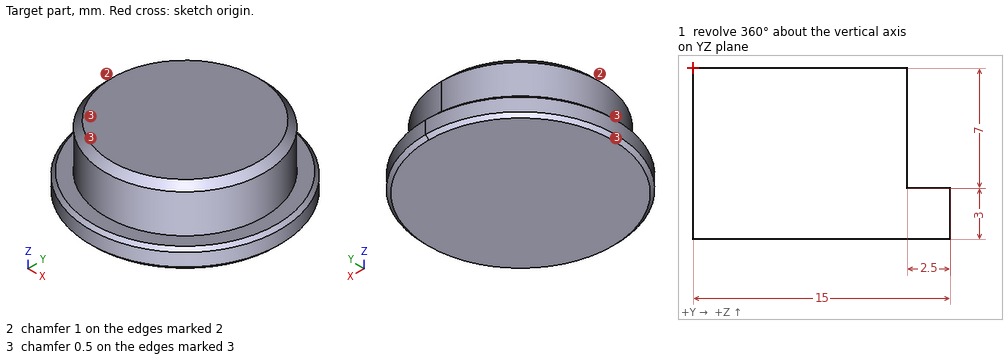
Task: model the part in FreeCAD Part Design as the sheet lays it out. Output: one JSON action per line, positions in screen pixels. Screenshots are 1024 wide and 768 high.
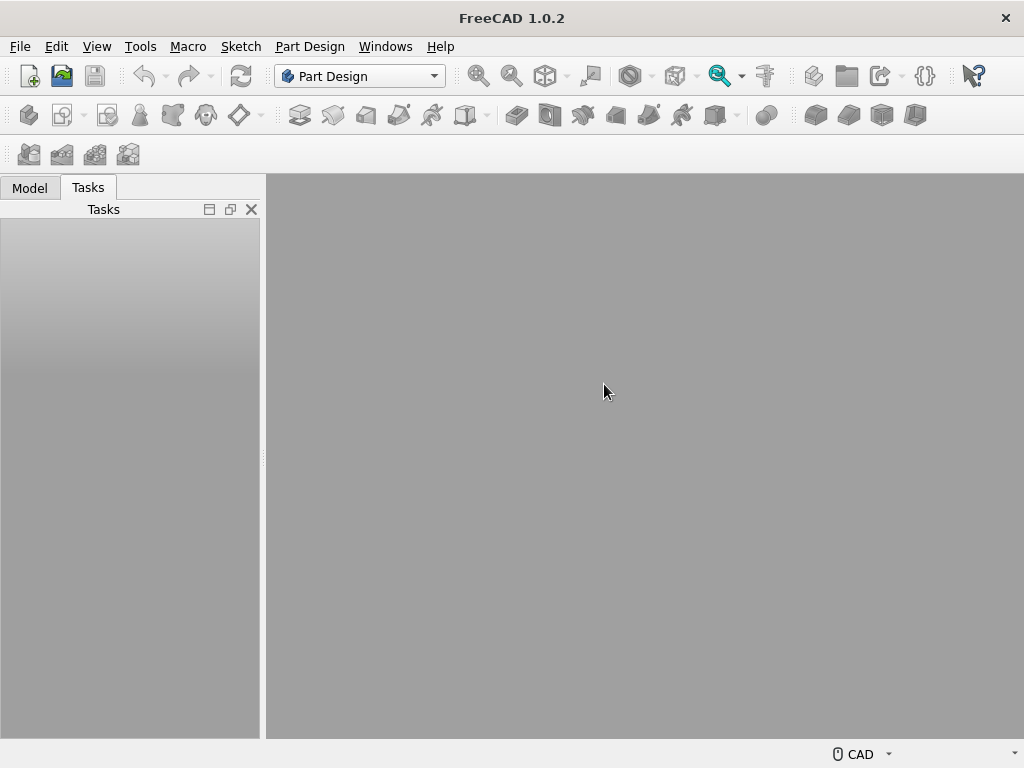
{"action": "left_click", "coordinate": [29, 76]}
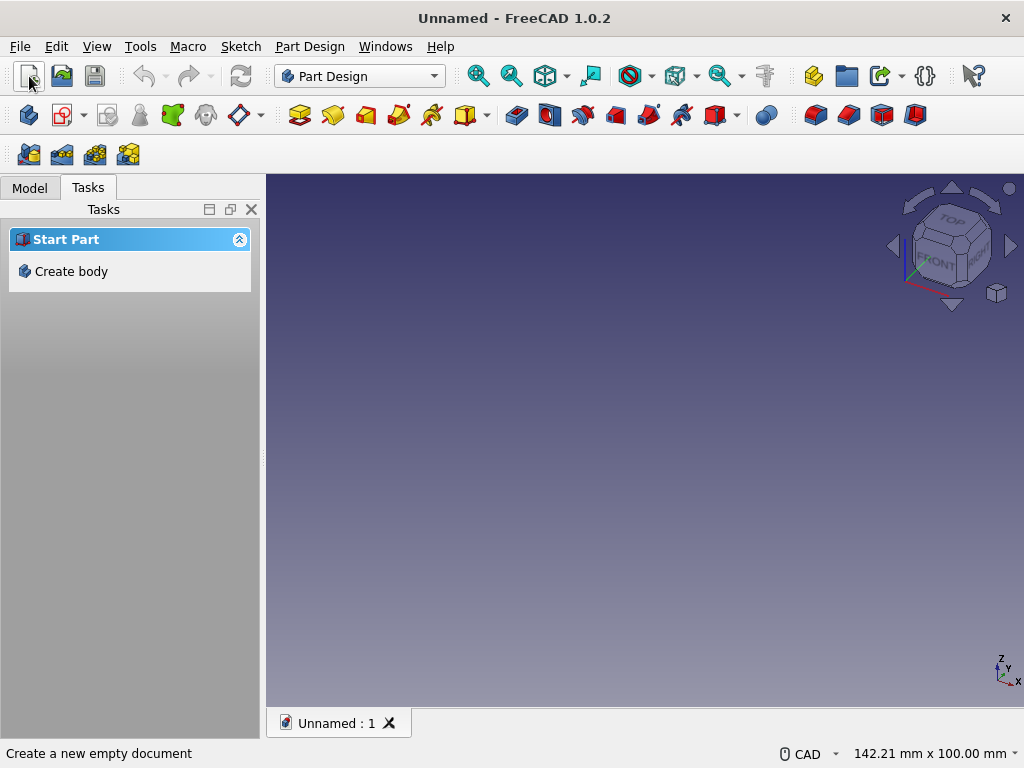
{"action": "left_click", "coordinate": [62, 116]}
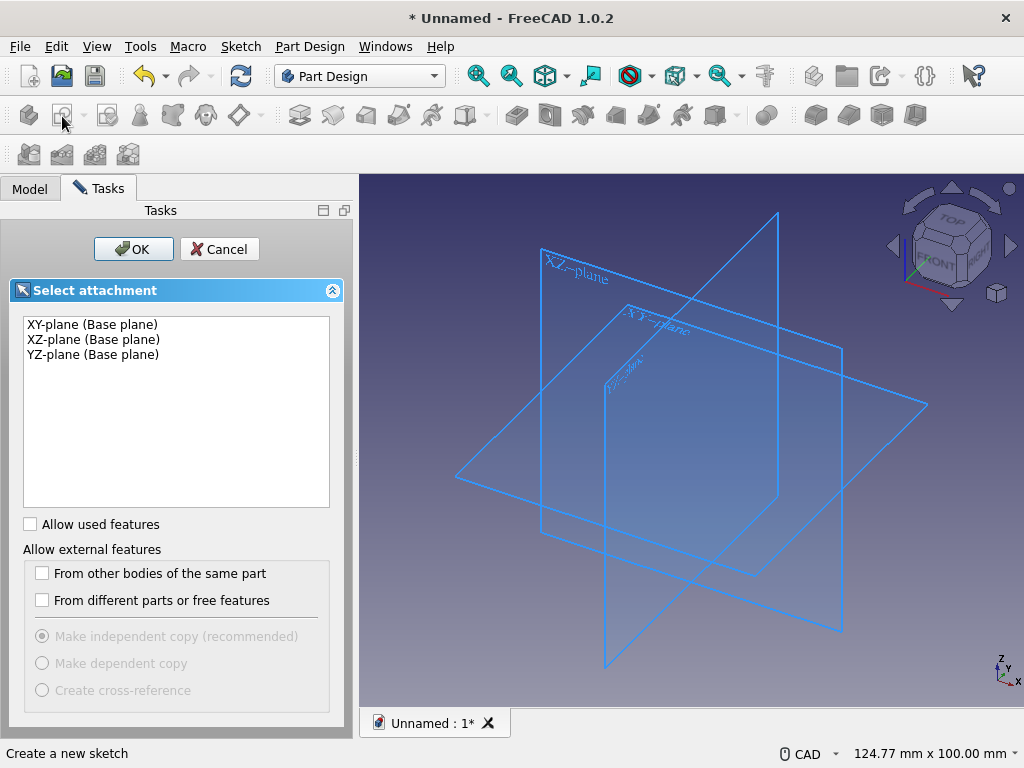
{"action": "left_click", "coordinate": [84, 354]}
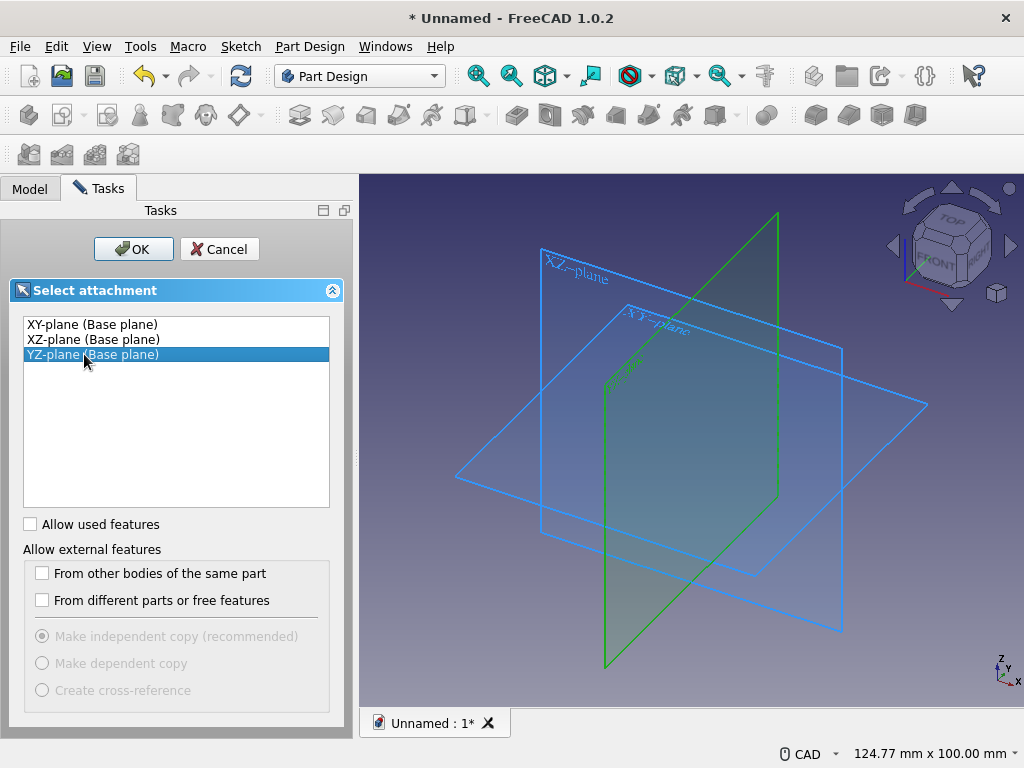
{"action": "left_click", "coordinate": [134, 249]}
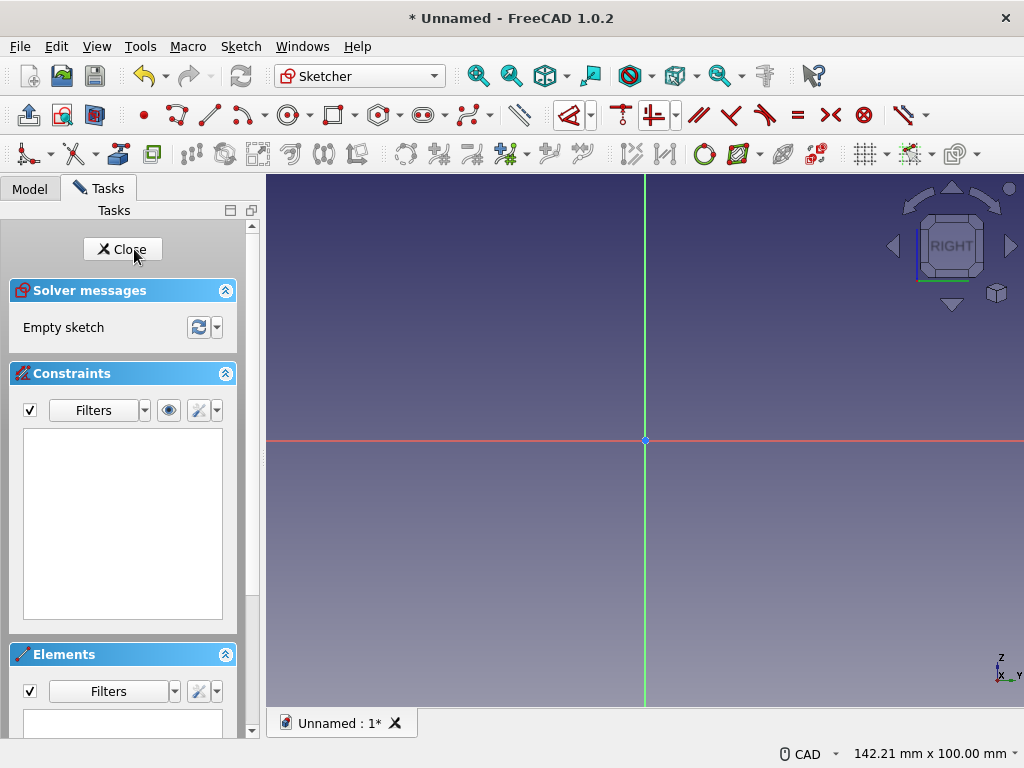
{"action": "scroll", "coordinate": [712, 474], "scroll_direction": "up", "scroll_amount": 8}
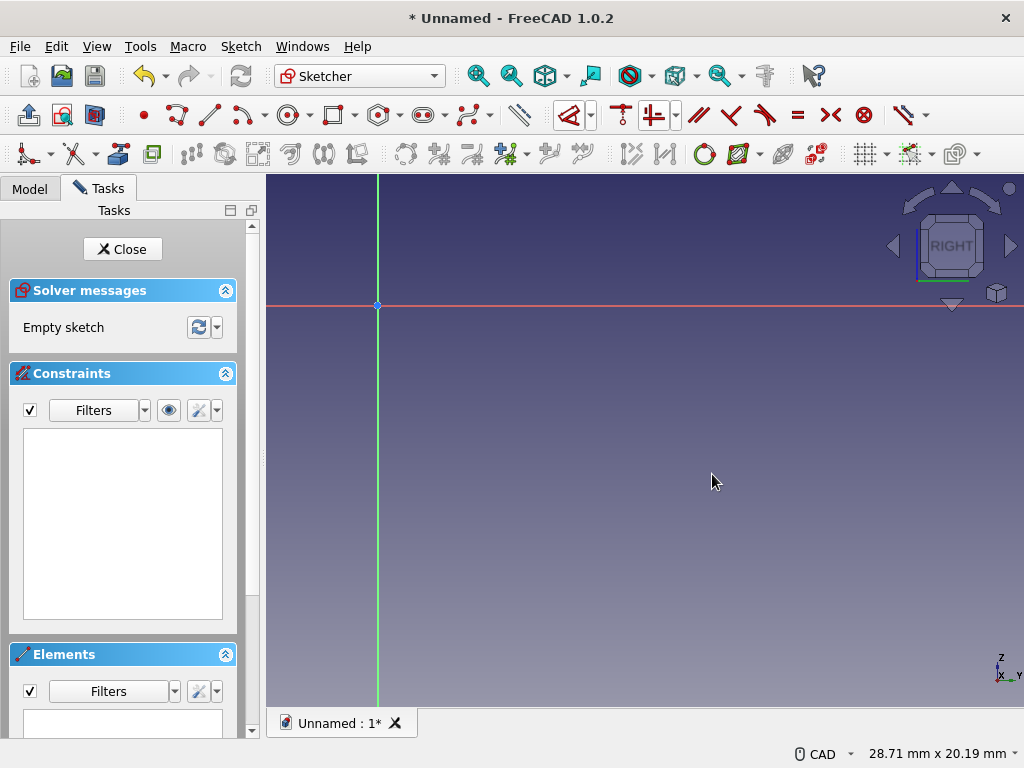
{"action": "left_click", "coordinate": [177, 116]}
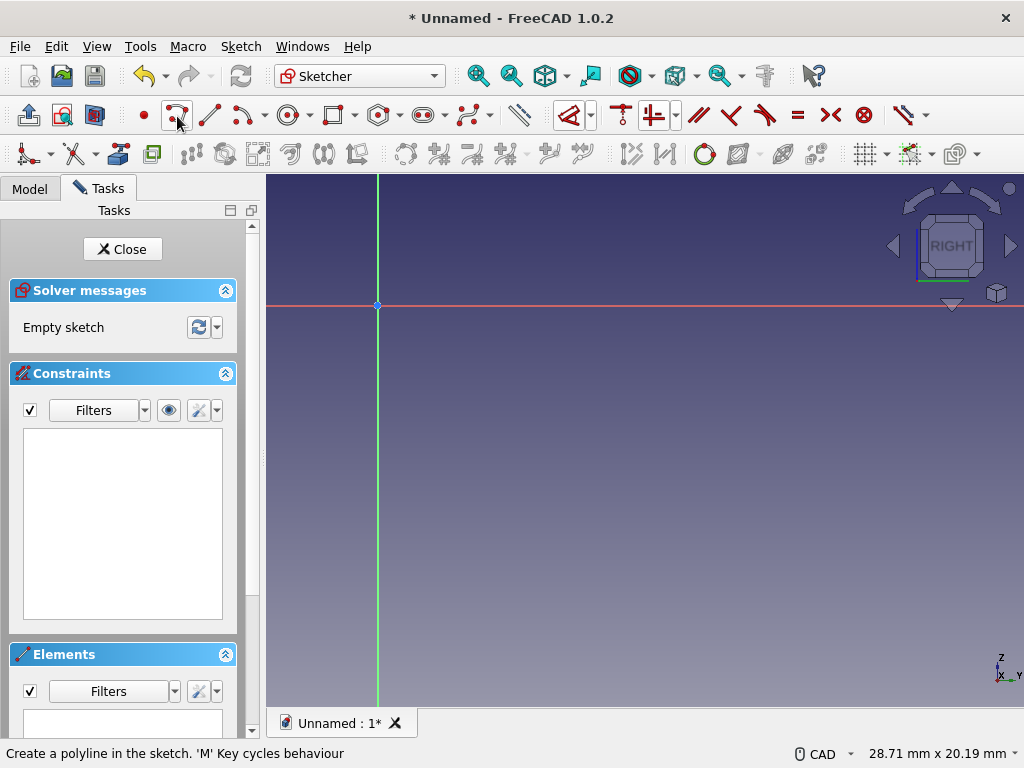
{"action": "left_click", "coordinate": [378, 306]}
{"action": "left_click", "coordinate": [387, 570]}
{"action": "left_click", "coordinate": [774, 570]}
{"action": "left_click", "coordinate": [774, 491]}
{"action": "left_click", "coordinate": [708, 491]}
{"action": "left_click", "coordinate": [708, 315]}
{"action": "left_click", "coordinate": [378, 306]}
{"action": "key", "text": "Escape"}
{"action": "key", "text": "Escape"}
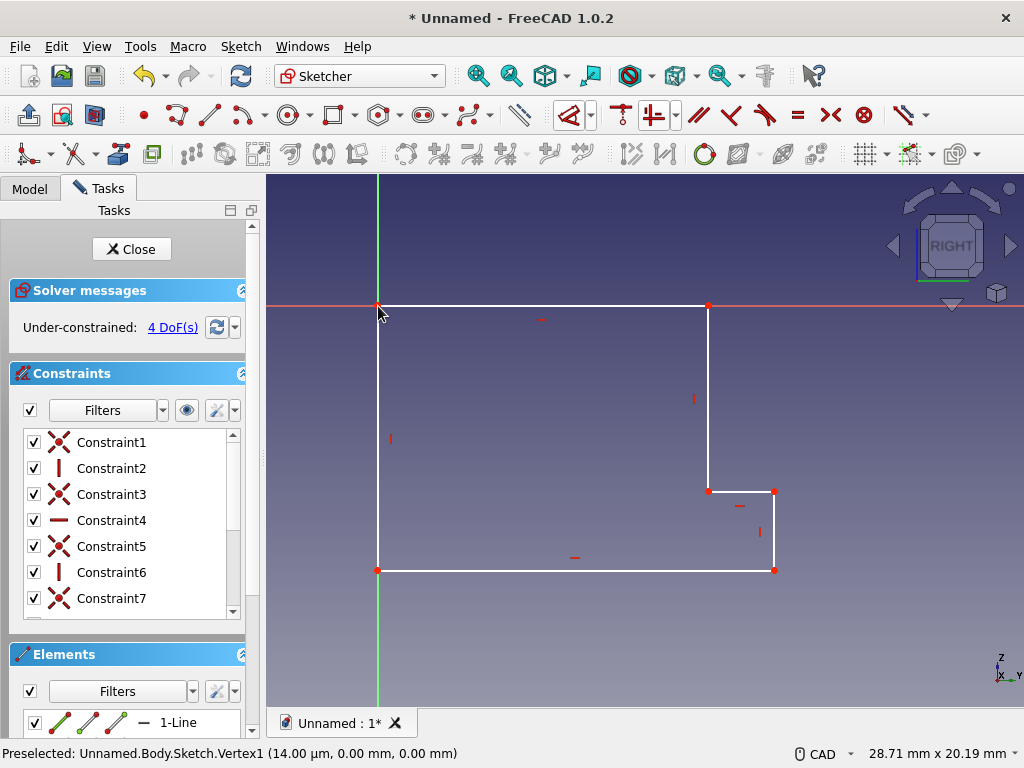
{"action": "left_click", "coordinate": [568, 116]}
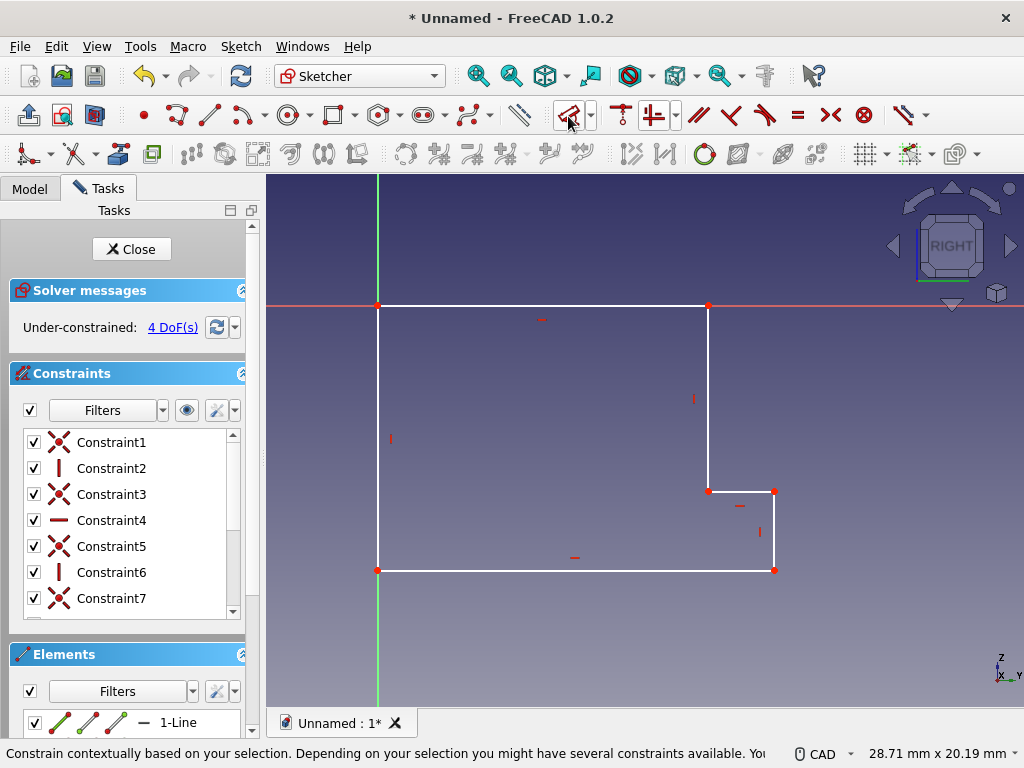
{"action": "left_click", "coordinate": [774, 547]}
{"action": "left_click", "coordinate": [808, 531]}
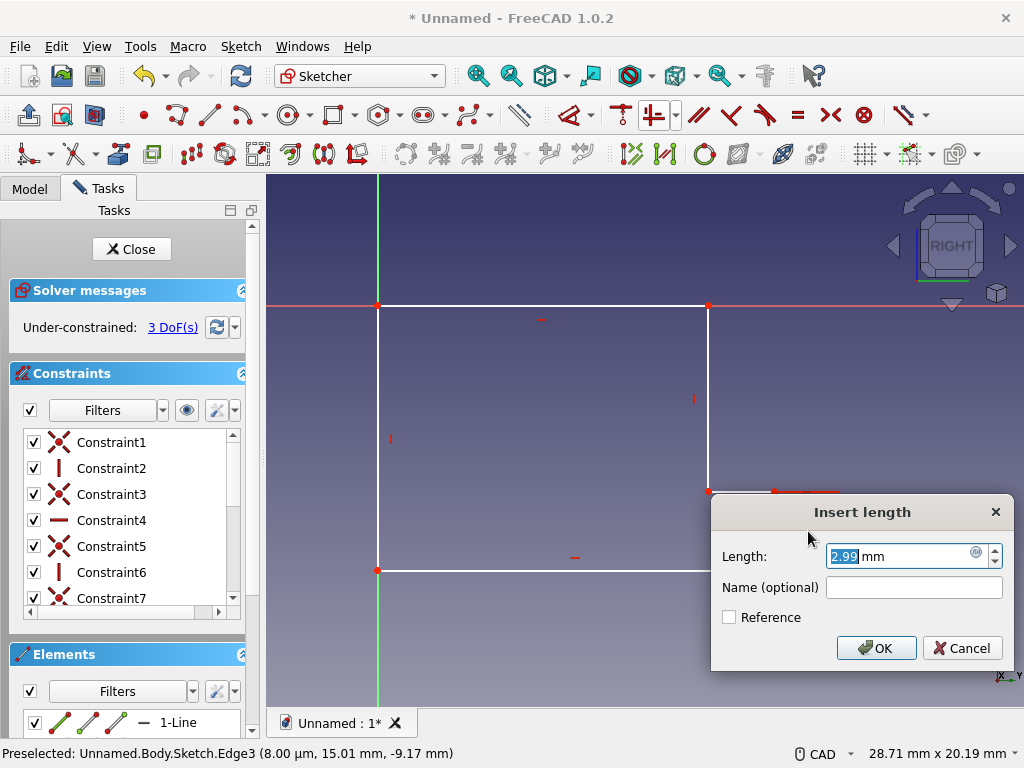
{"action": "type", "text": "3"}
{"action": "key", "text": "Return"}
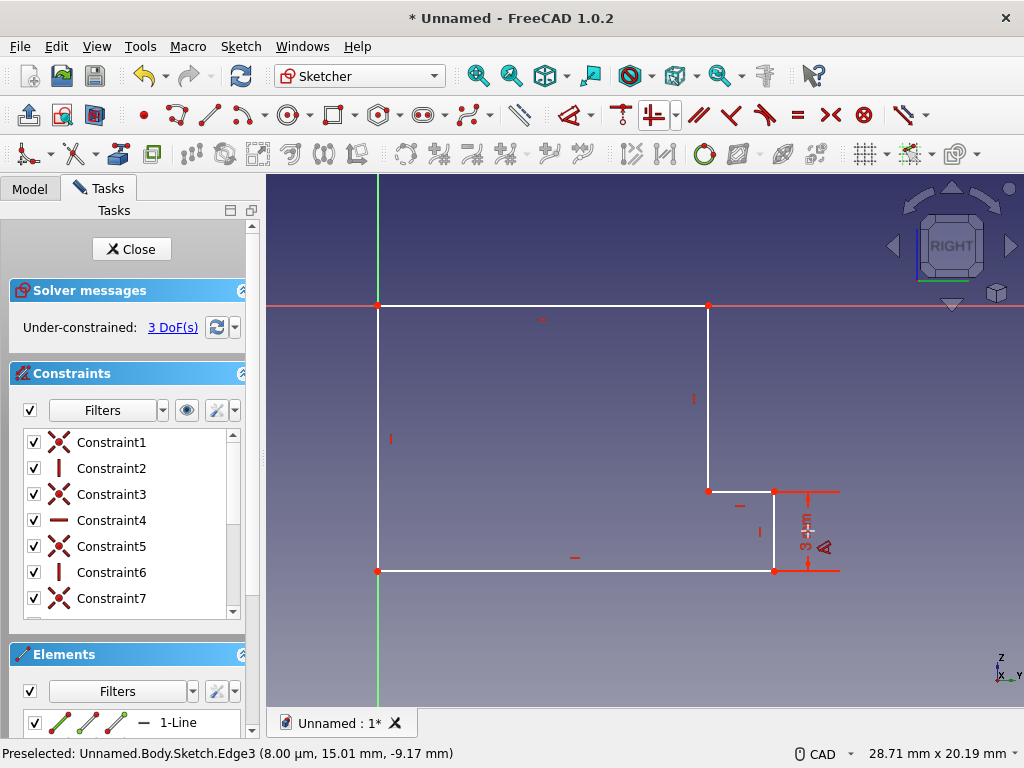
{"action": "left_click", "coordinate": [708, 436]}
{"action": "left_click", "coordinate": [742, 399]}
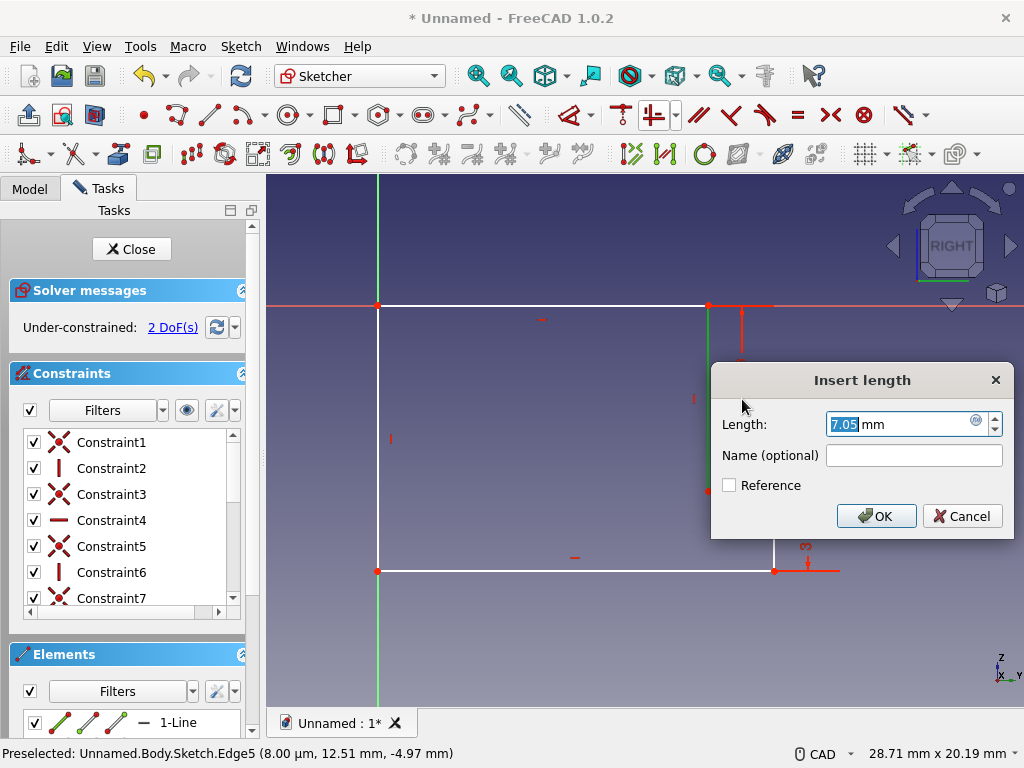
{"action": "type", "text": "7"}
{"action": "key", "text": "Return"}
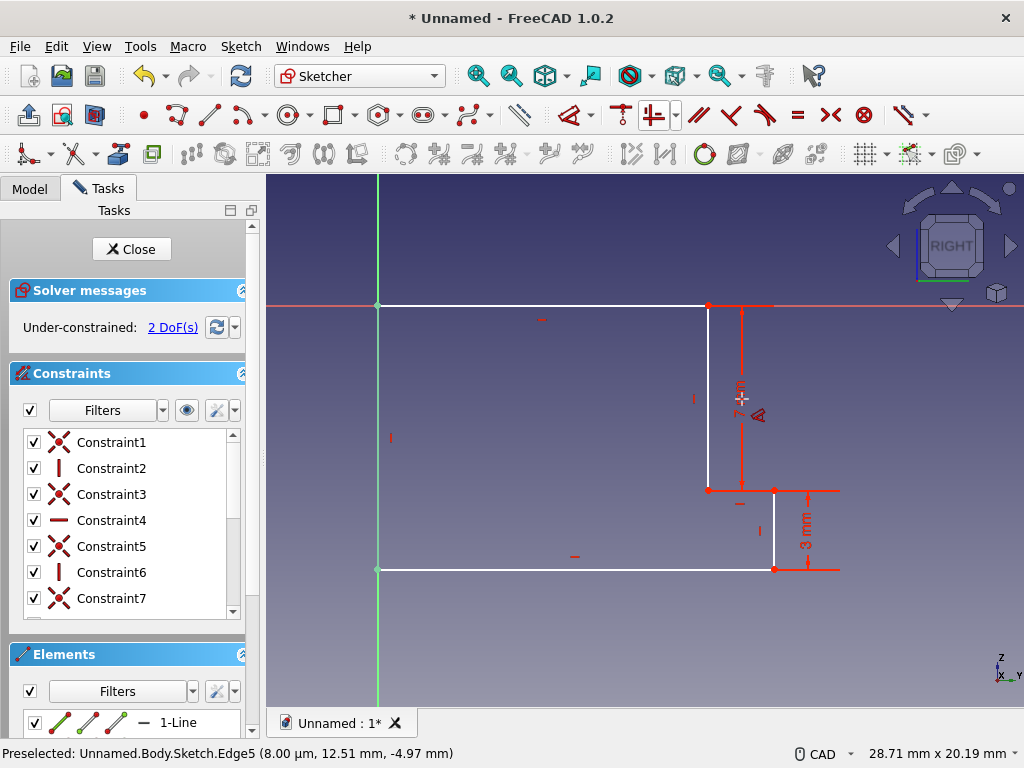
{"action": "left_click", "coordinate": [497, 570]}
{"action": "left_click", "coordinate": [576, 604]}